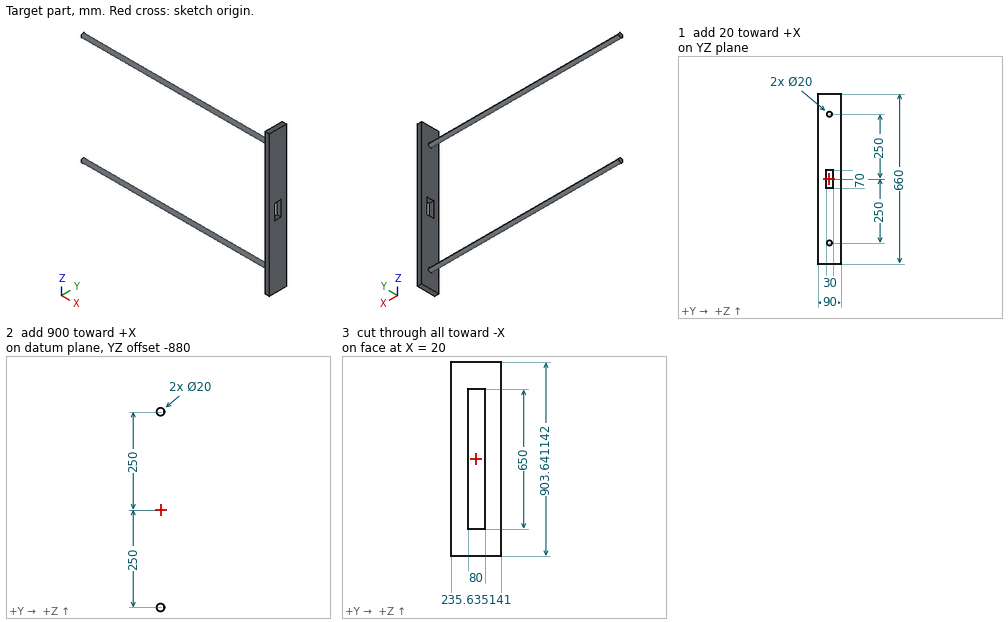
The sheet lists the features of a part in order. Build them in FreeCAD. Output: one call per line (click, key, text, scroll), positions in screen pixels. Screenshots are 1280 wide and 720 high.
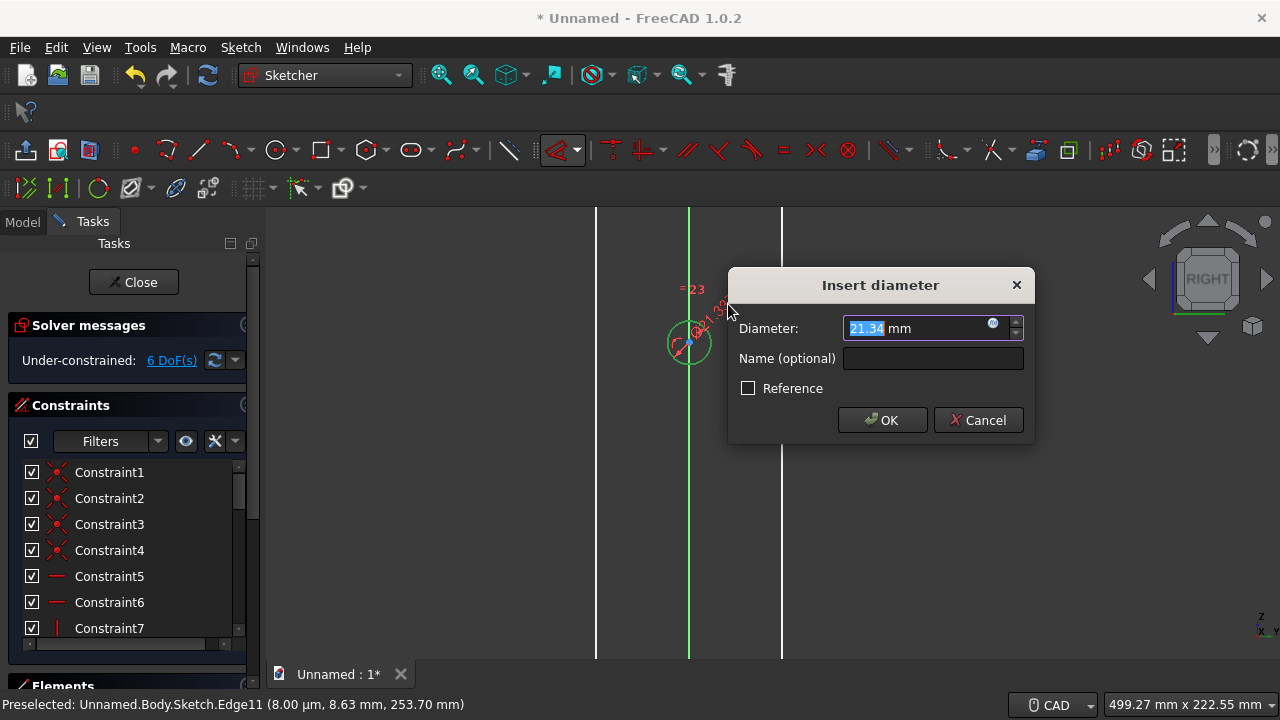
text(20)
key(Return)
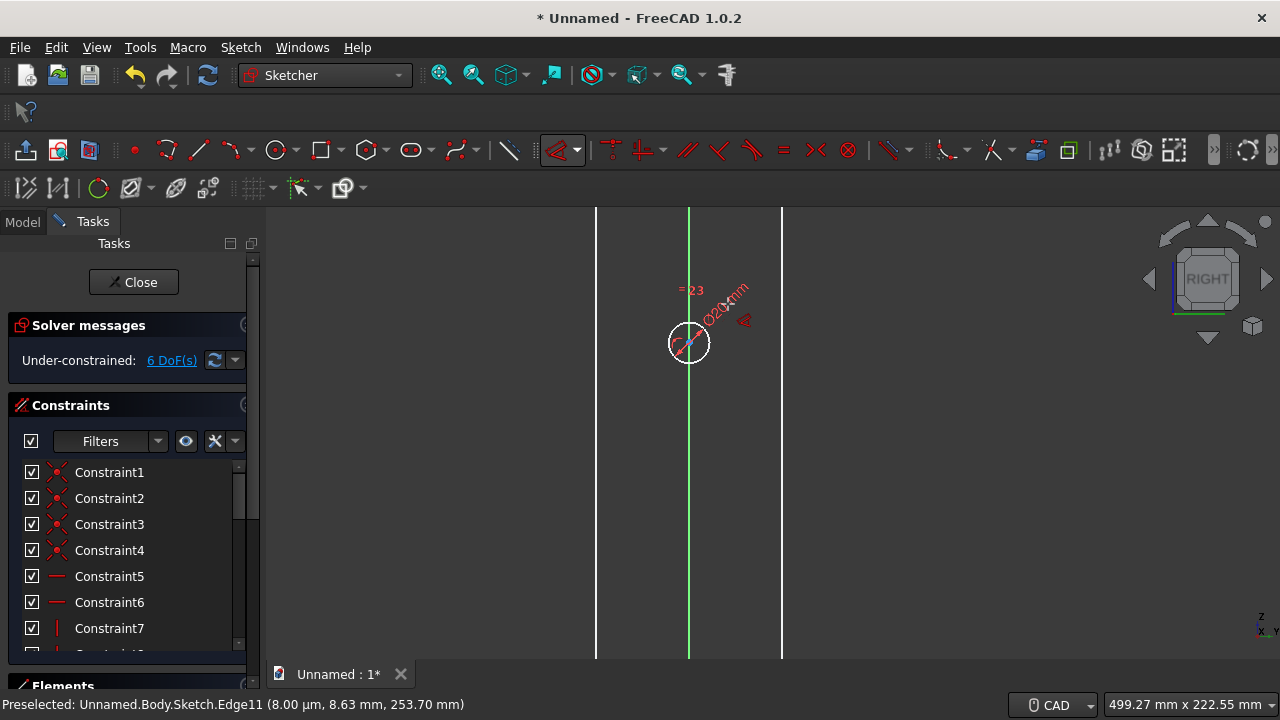
scroll(708, 329, down, 8)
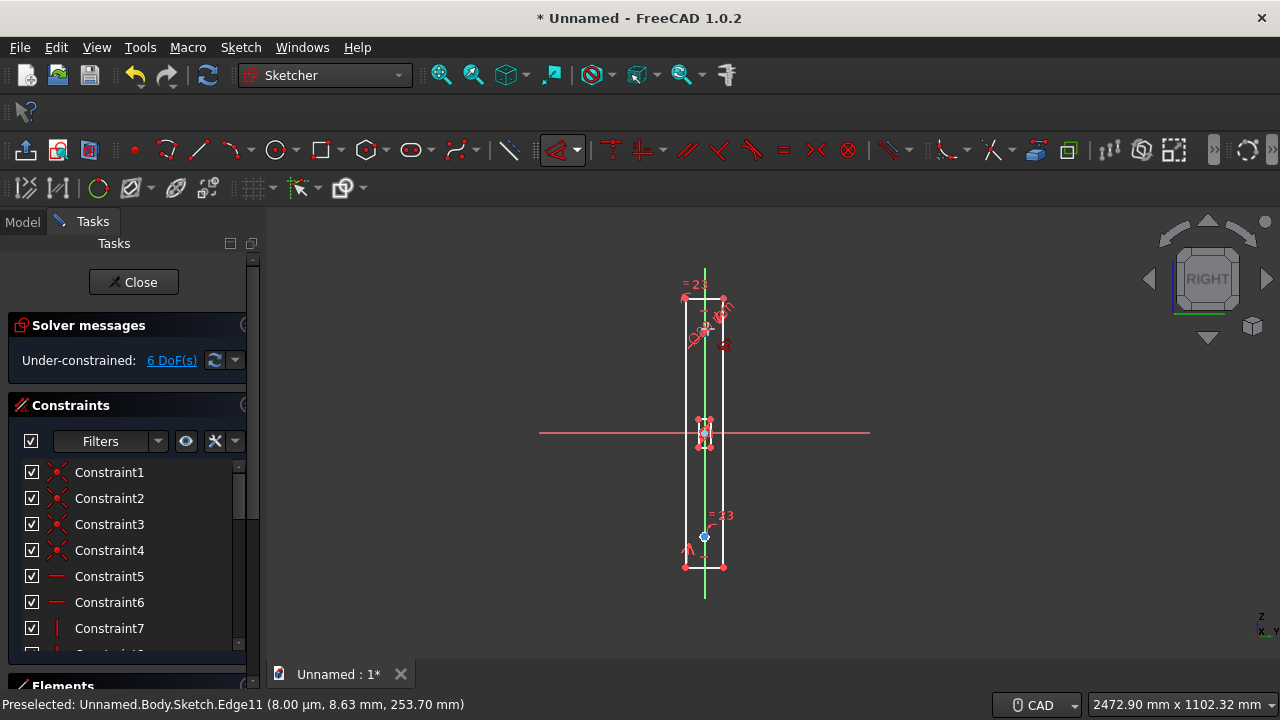
scroll(697, 568, up, 4)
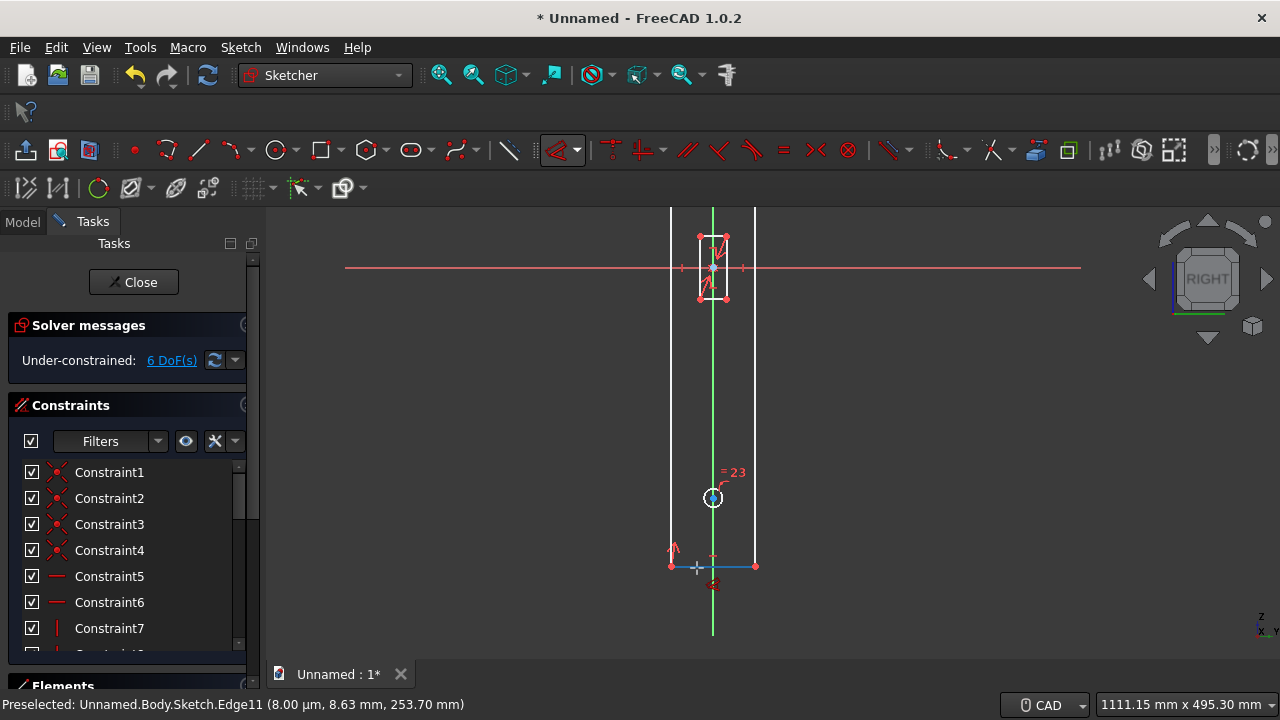
click(697, 567)
click(694, 601)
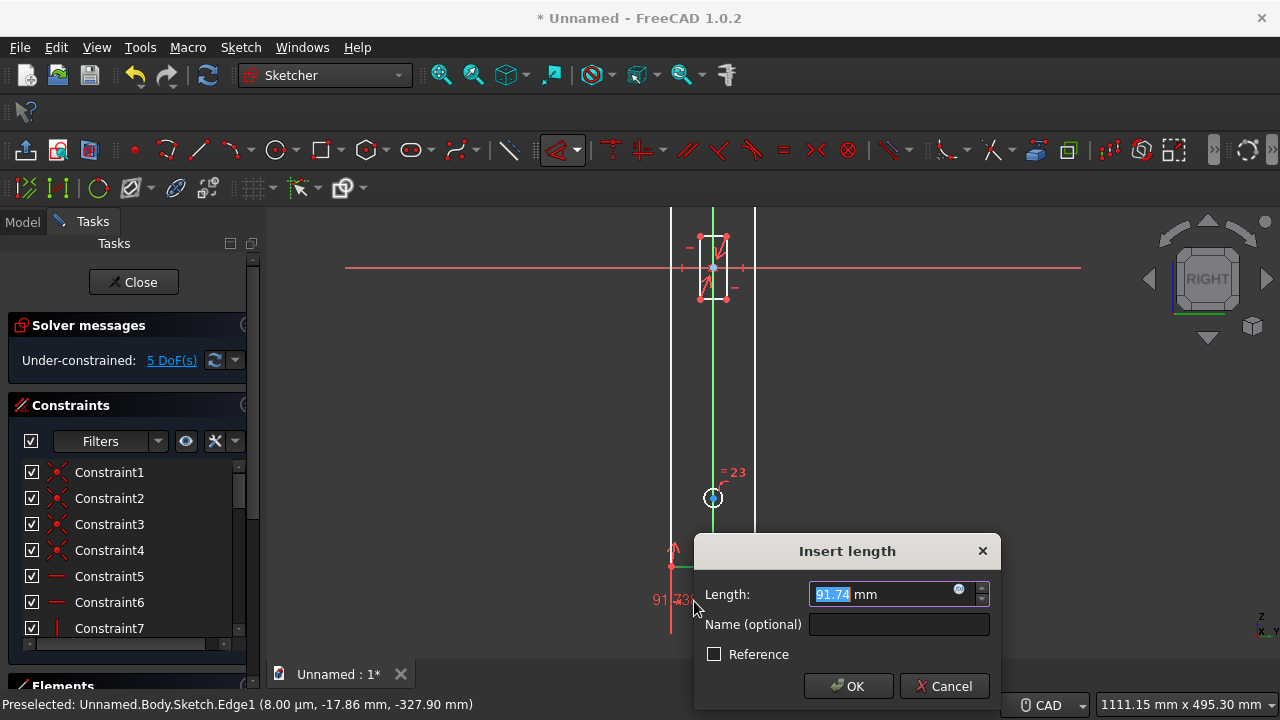
text(90)
key(Return)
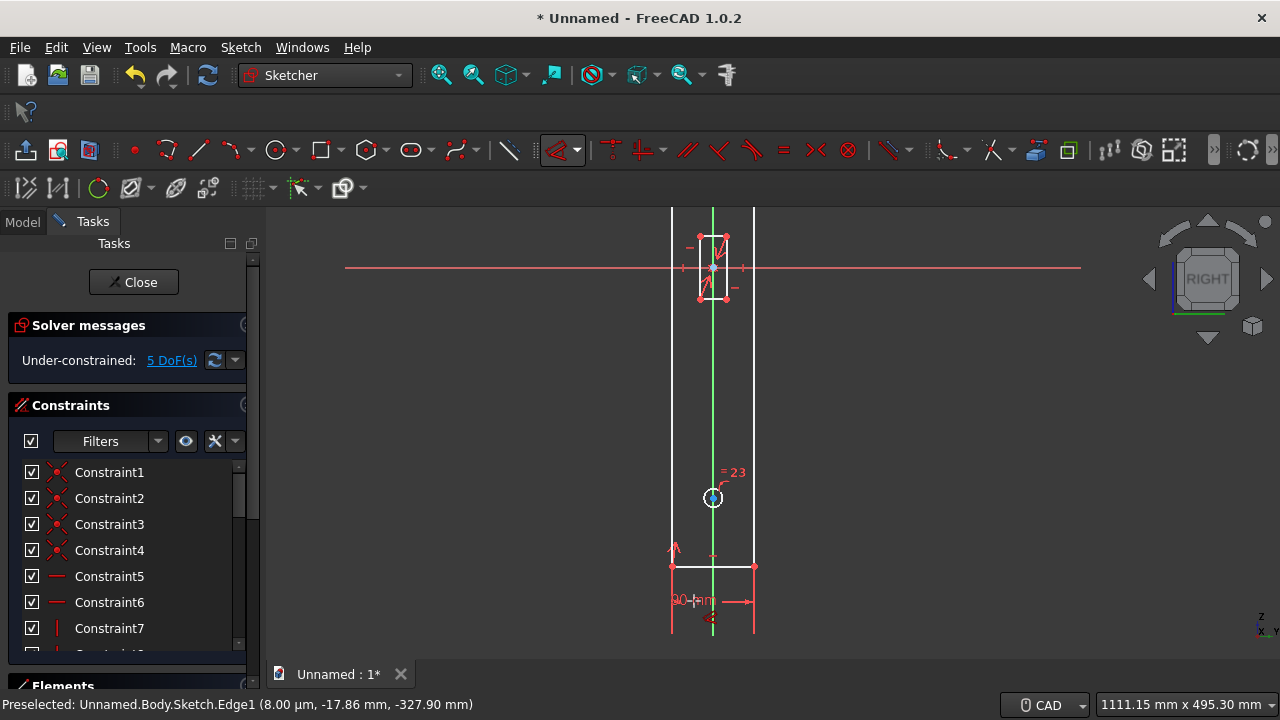
scroll(711, 299, up, 2)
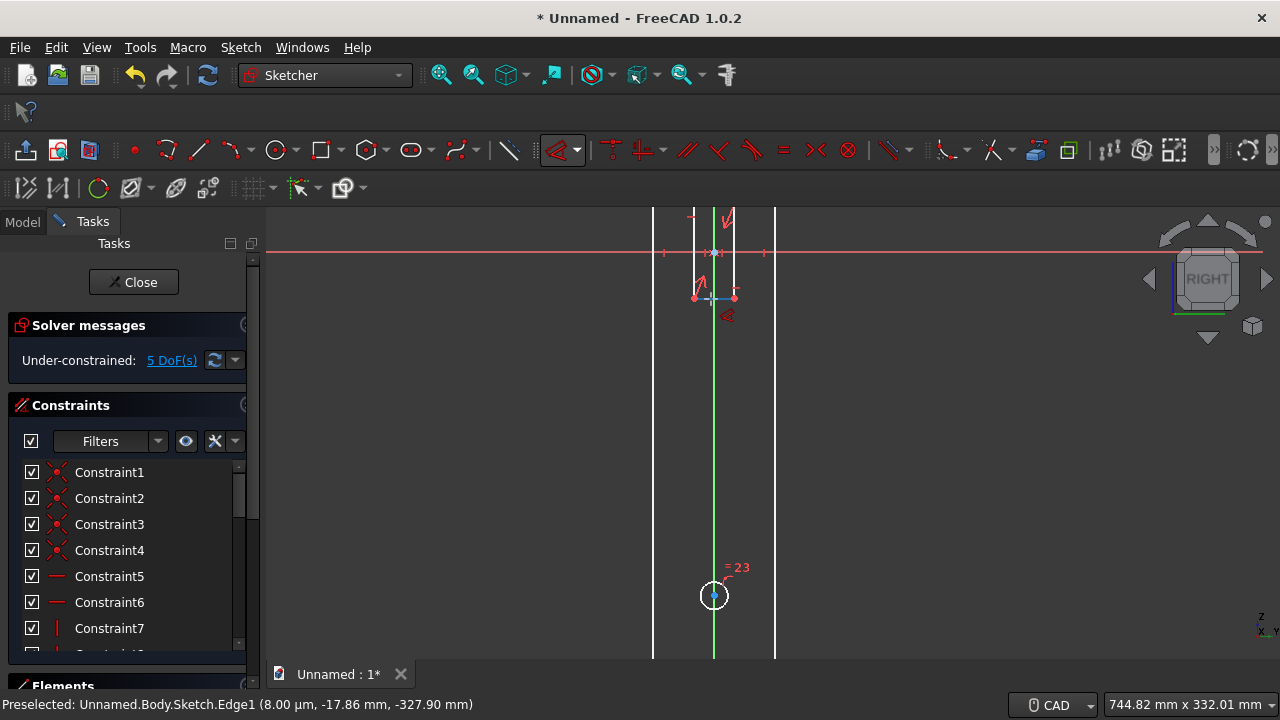
click(710, 299)
click(700, 333)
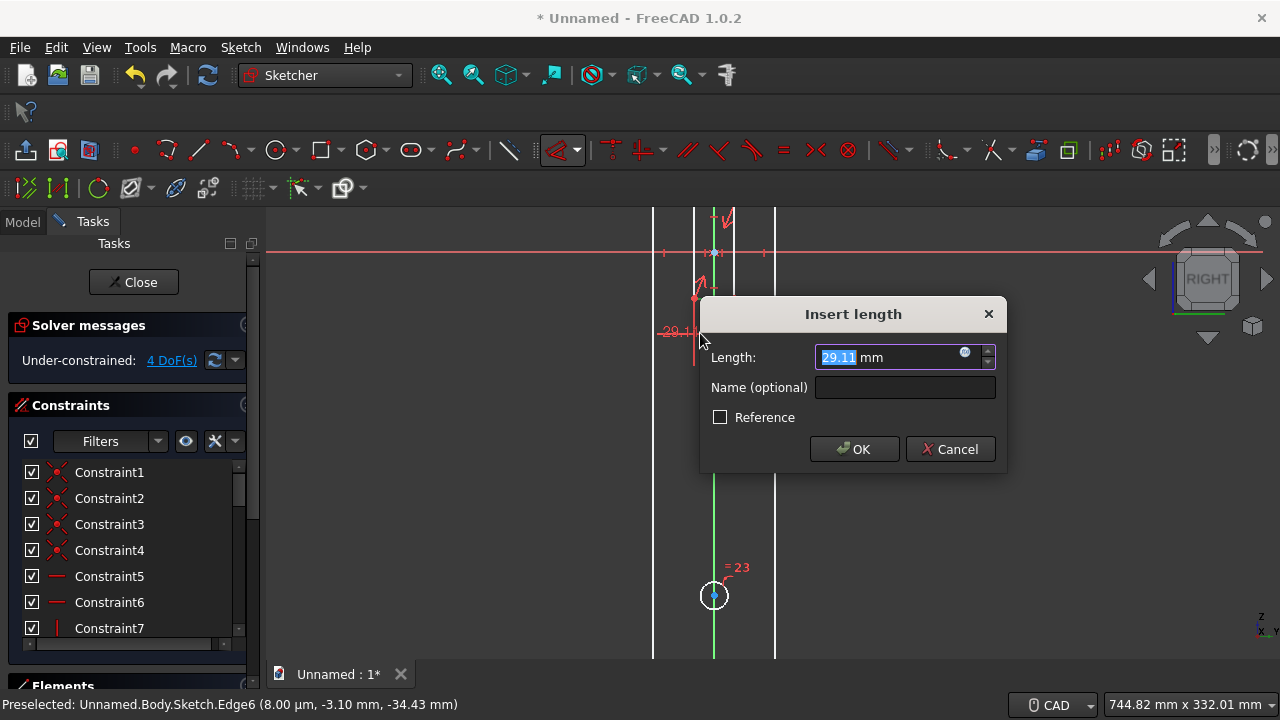
text(30)
key(Return)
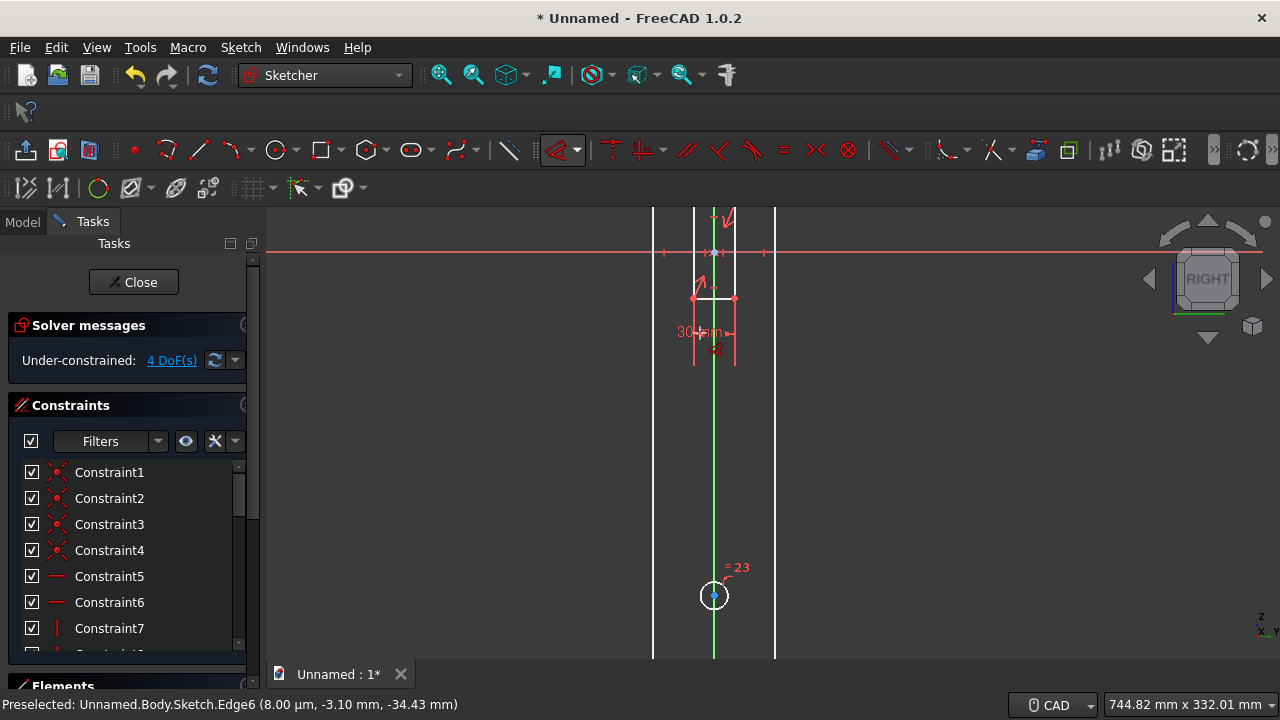
click(735, 271)
click(793, 267)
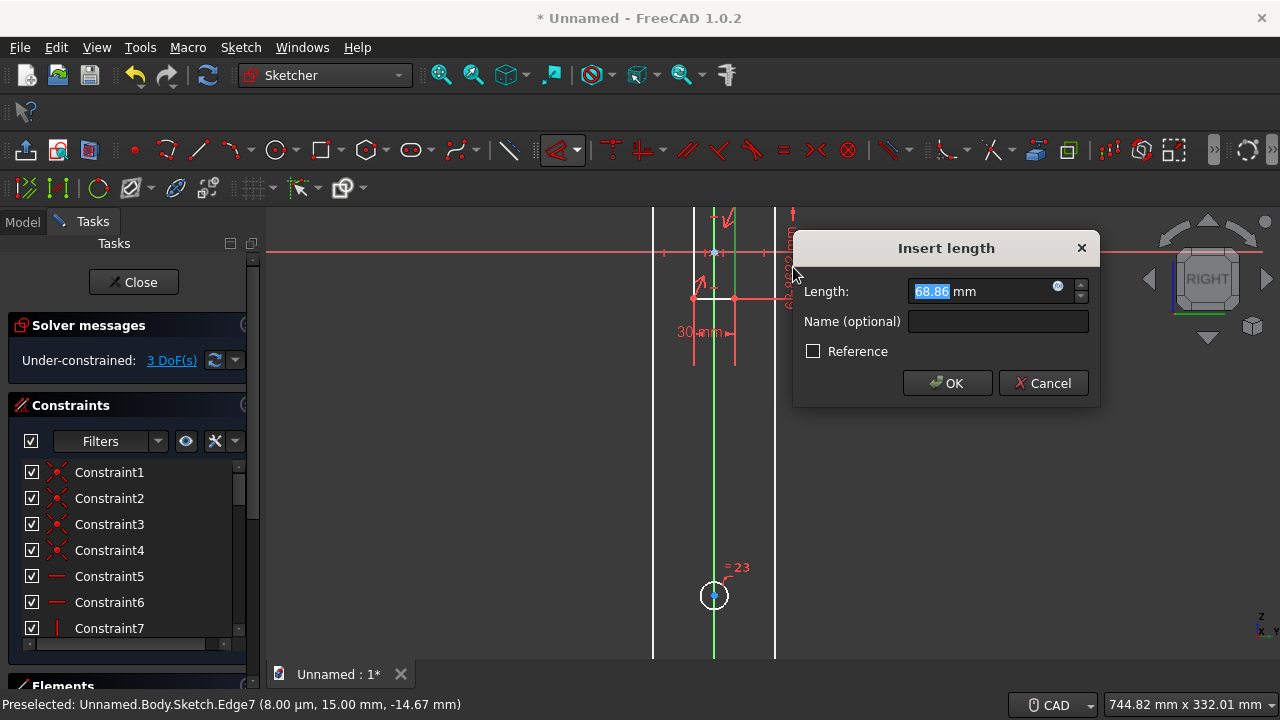
text(70)
key(Return)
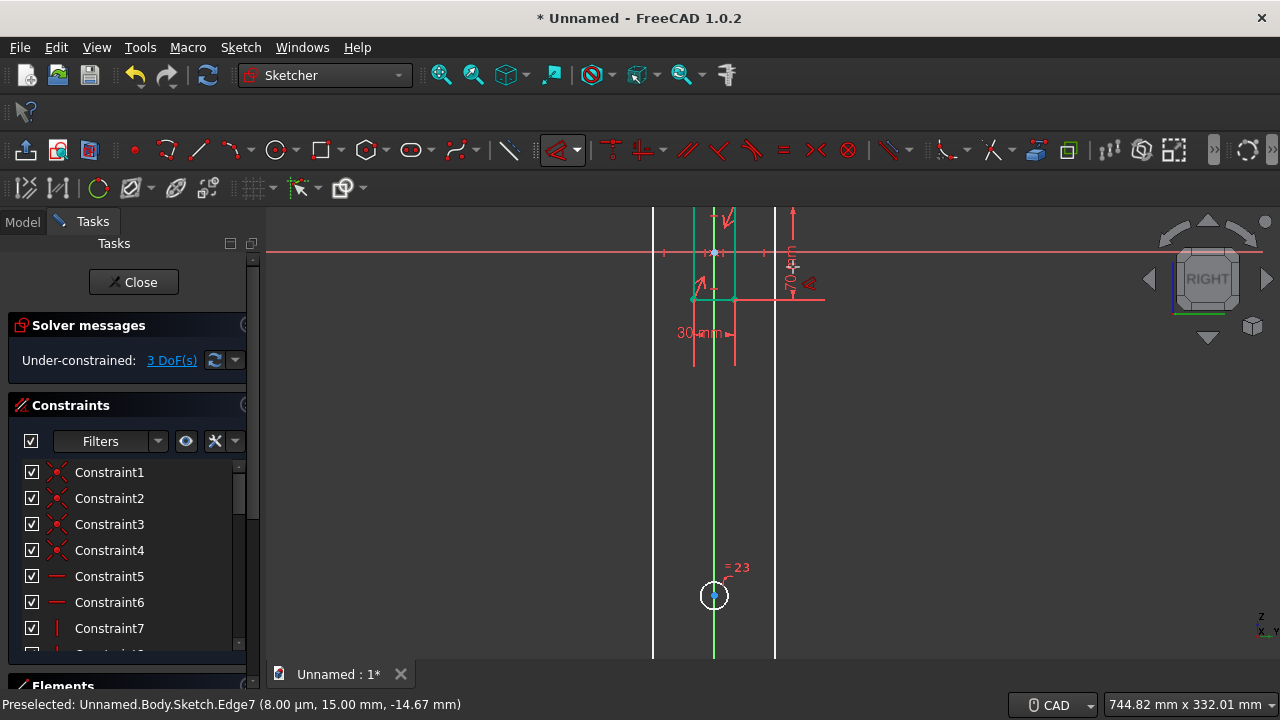
click(775, 431)
click(809, 433)